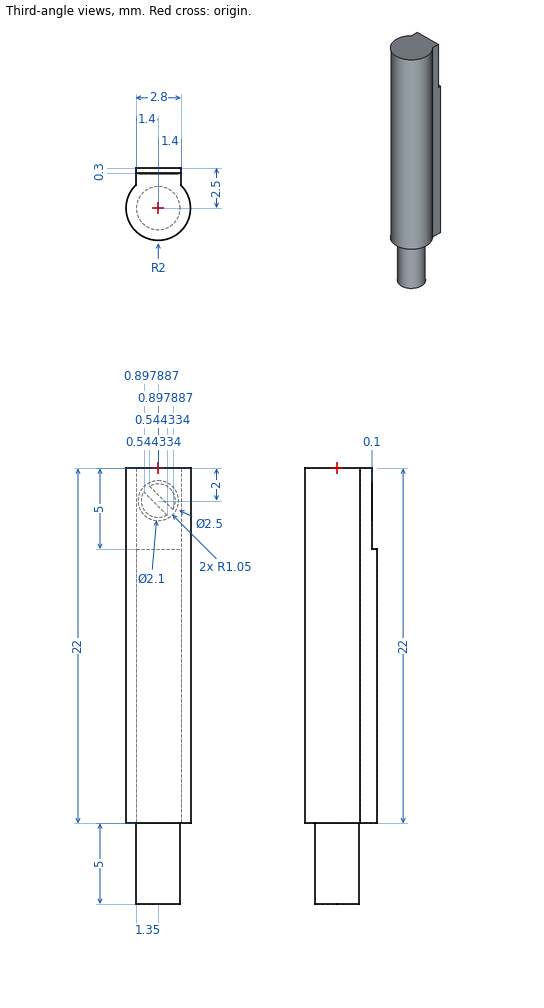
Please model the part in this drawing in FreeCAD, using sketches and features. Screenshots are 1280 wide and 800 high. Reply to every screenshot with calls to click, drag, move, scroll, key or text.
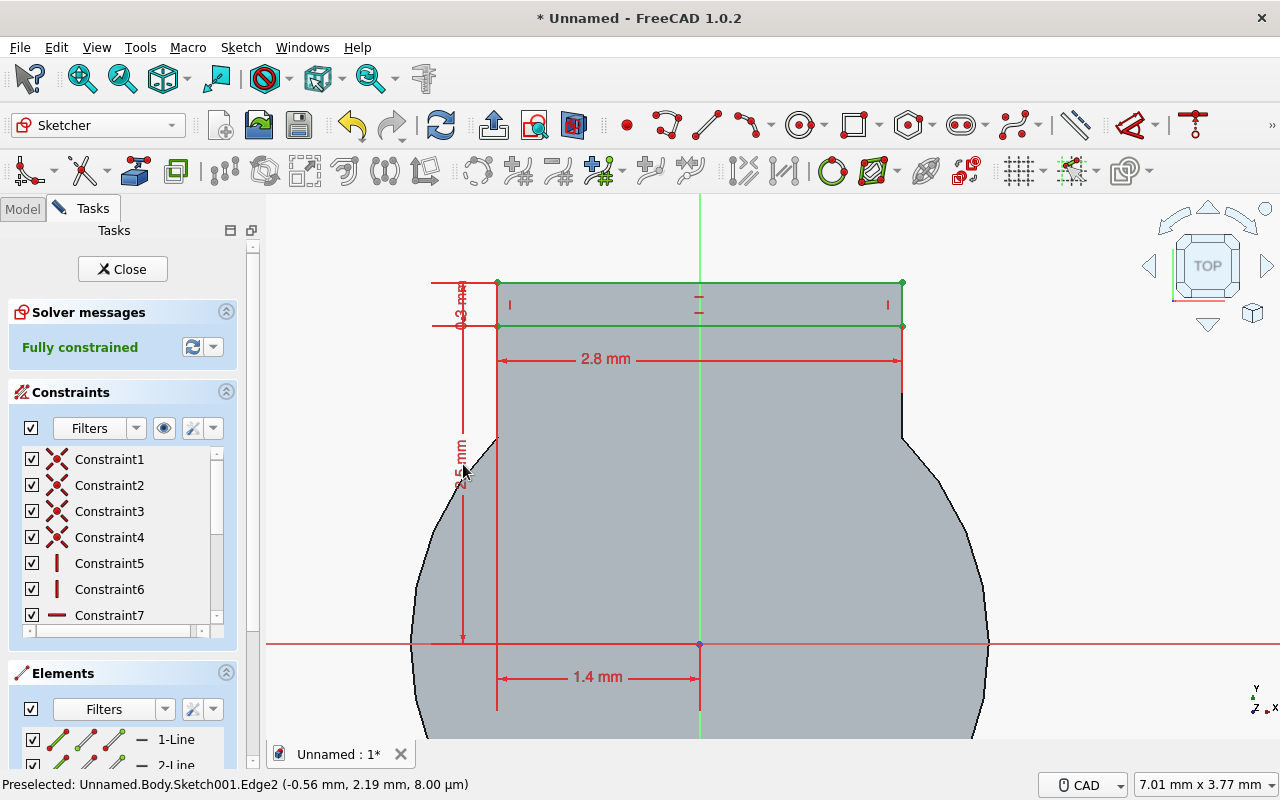
click(123, 269)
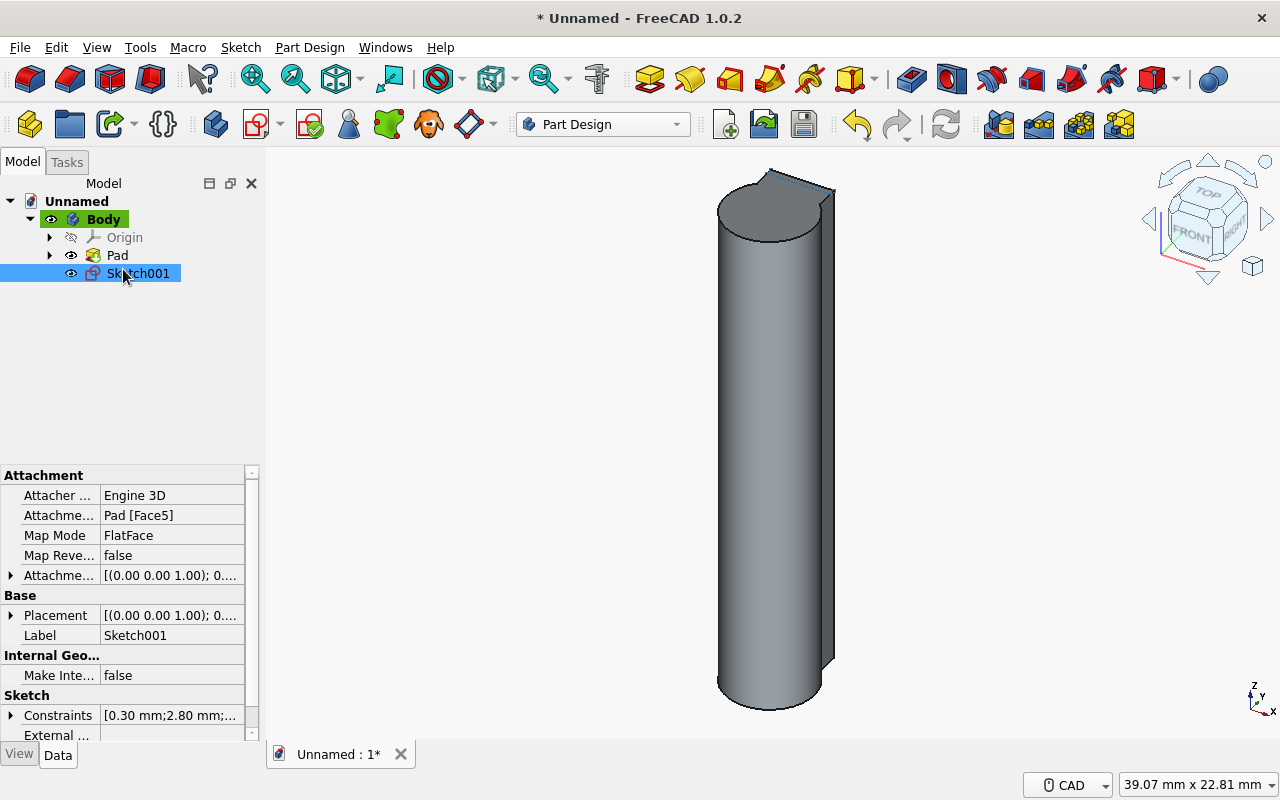
click(912, 80)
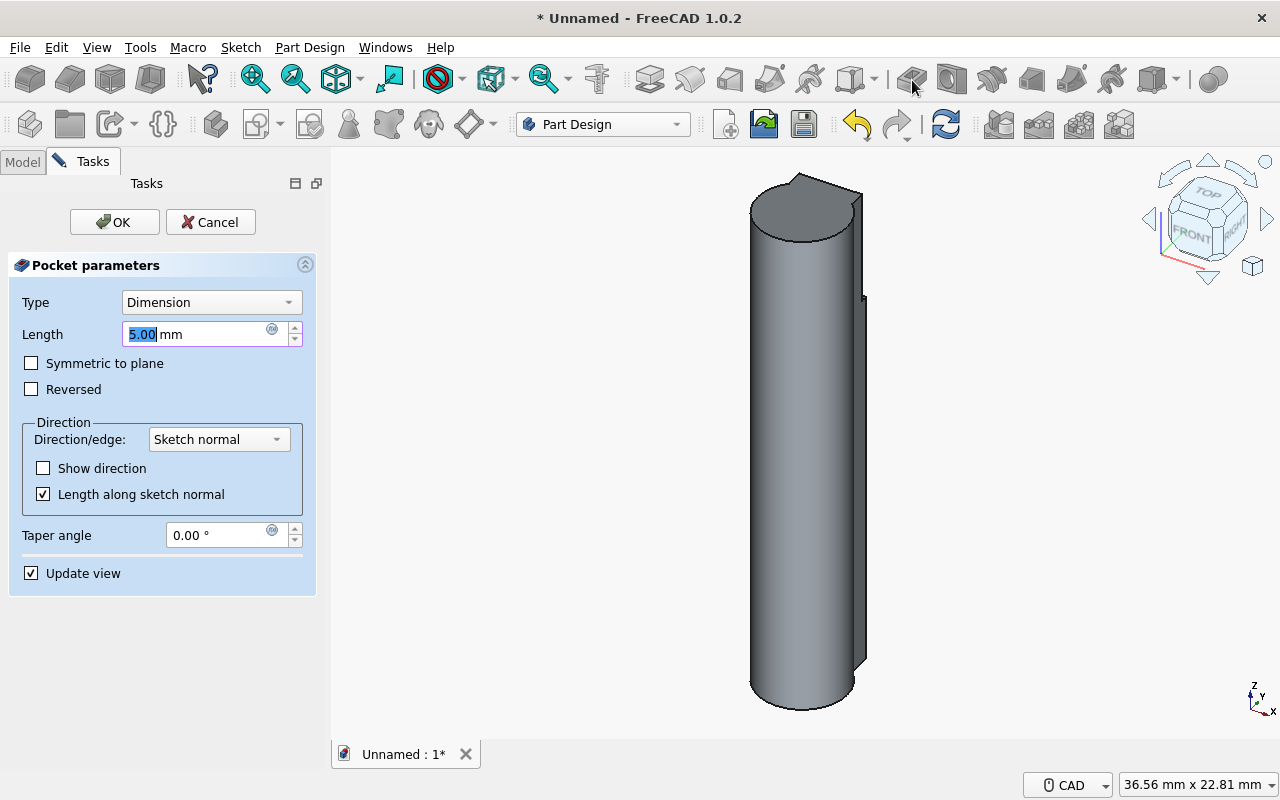
text(5)
key(Tab)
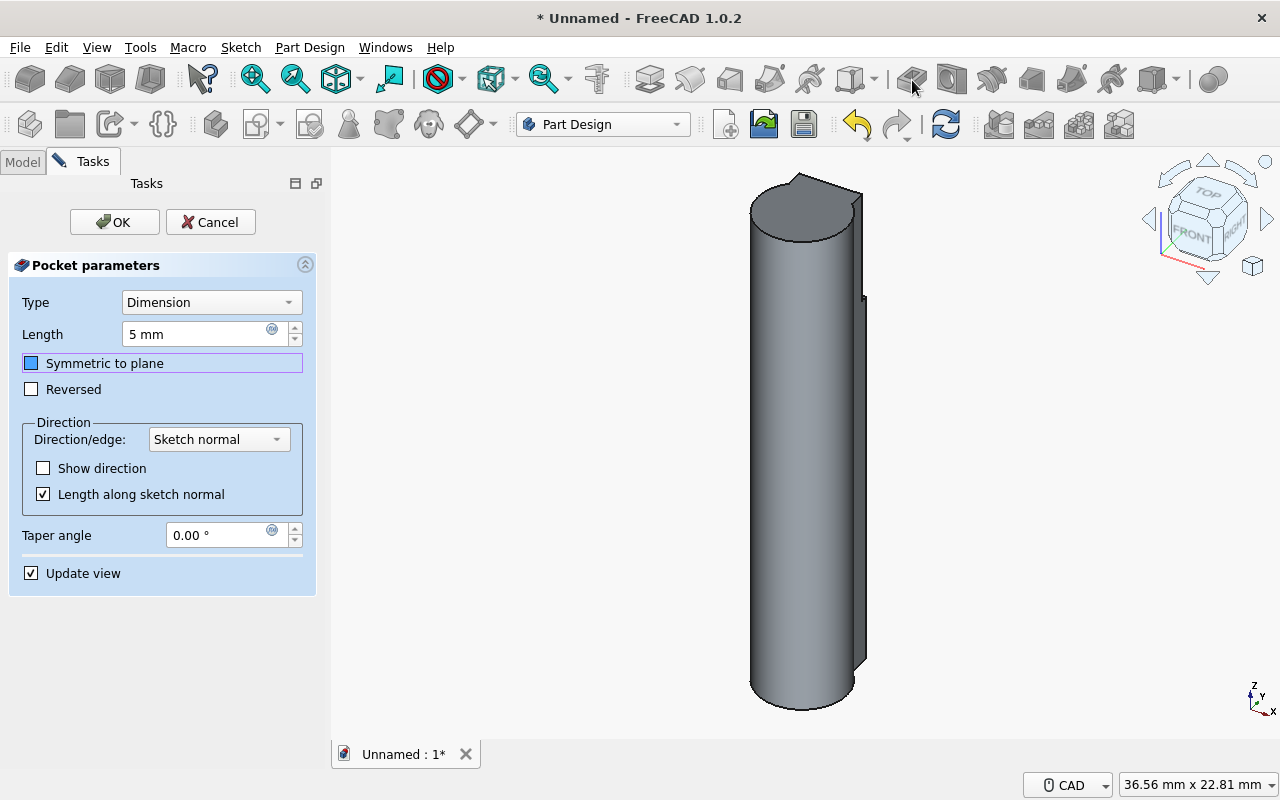
click(115, 222)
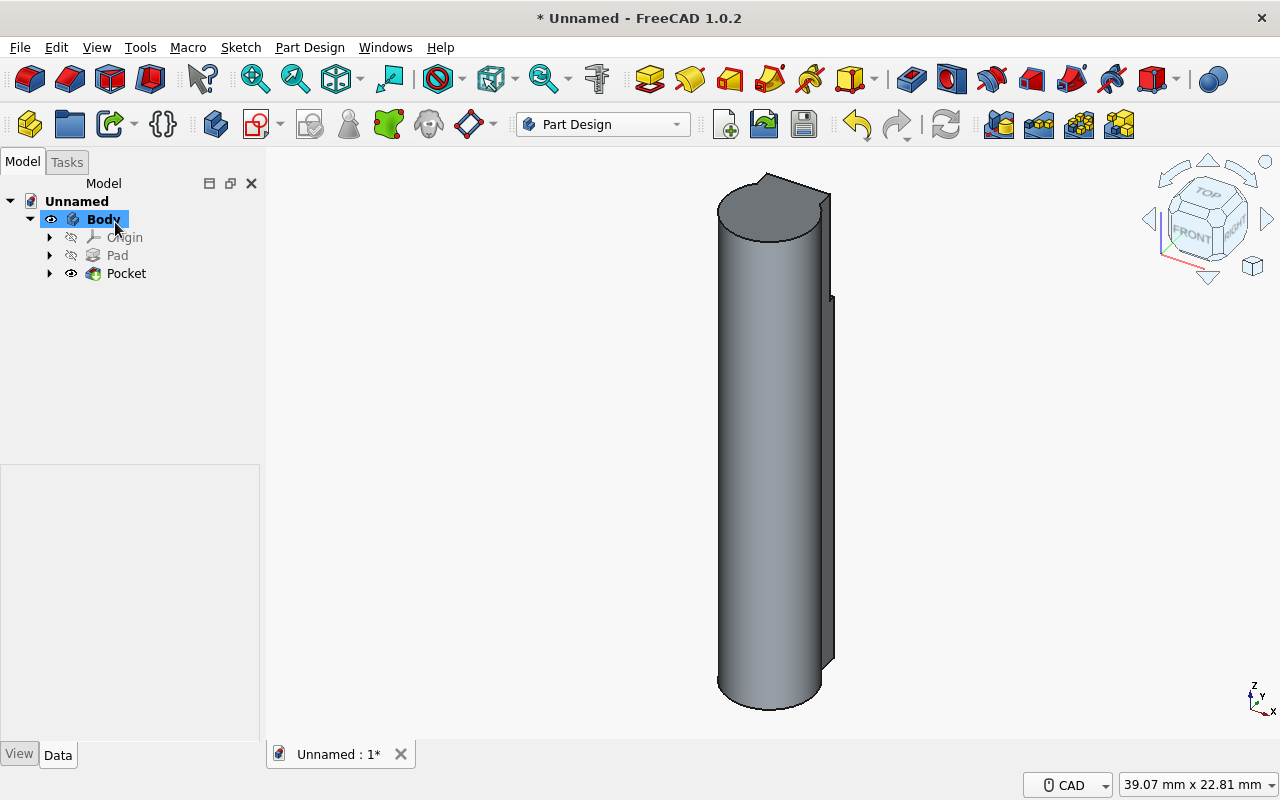
key(4)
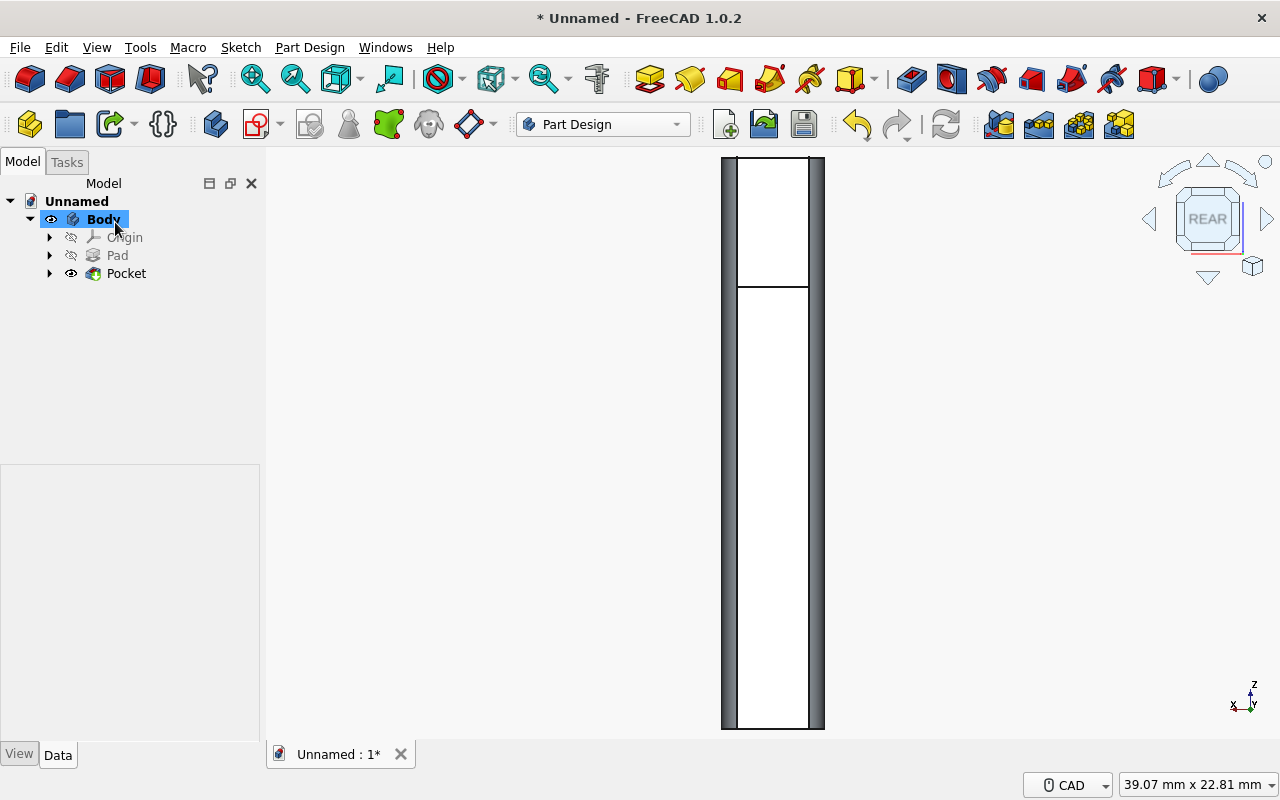
click(773, 203)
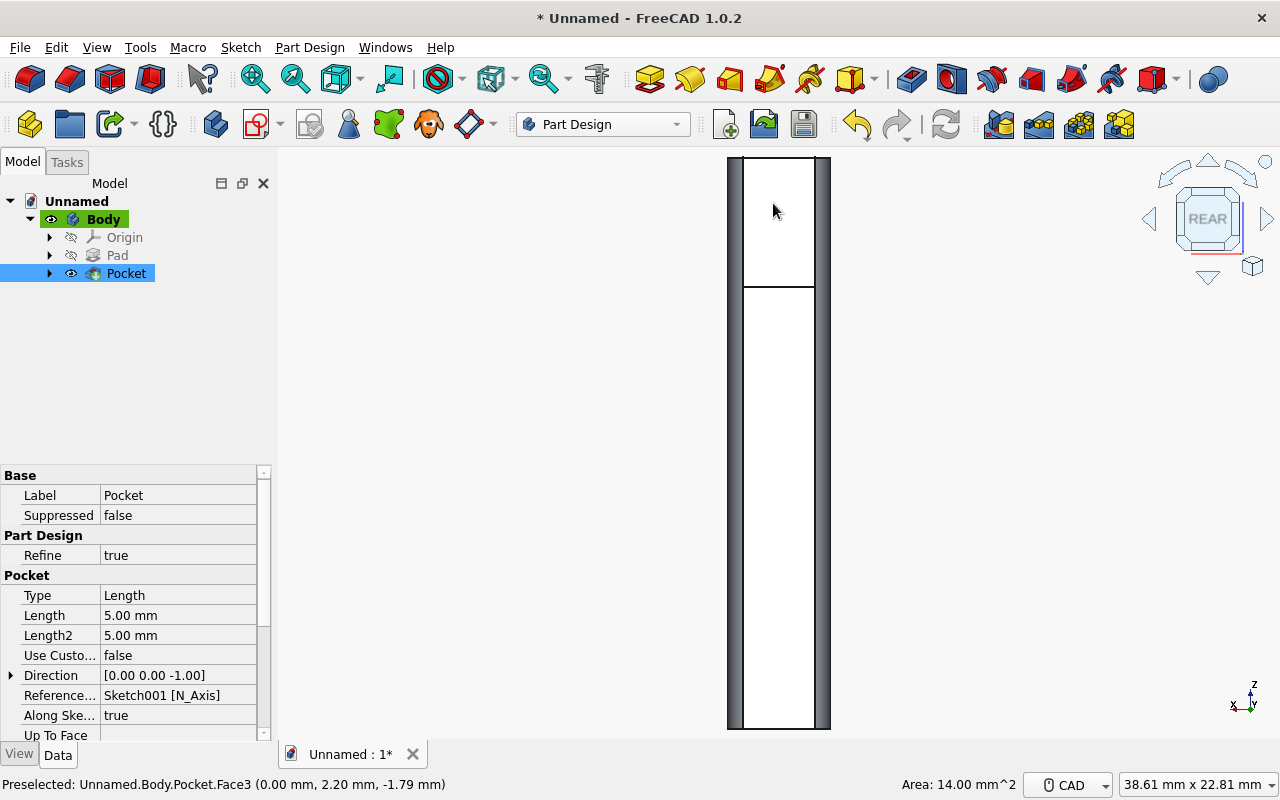
click(256, 124)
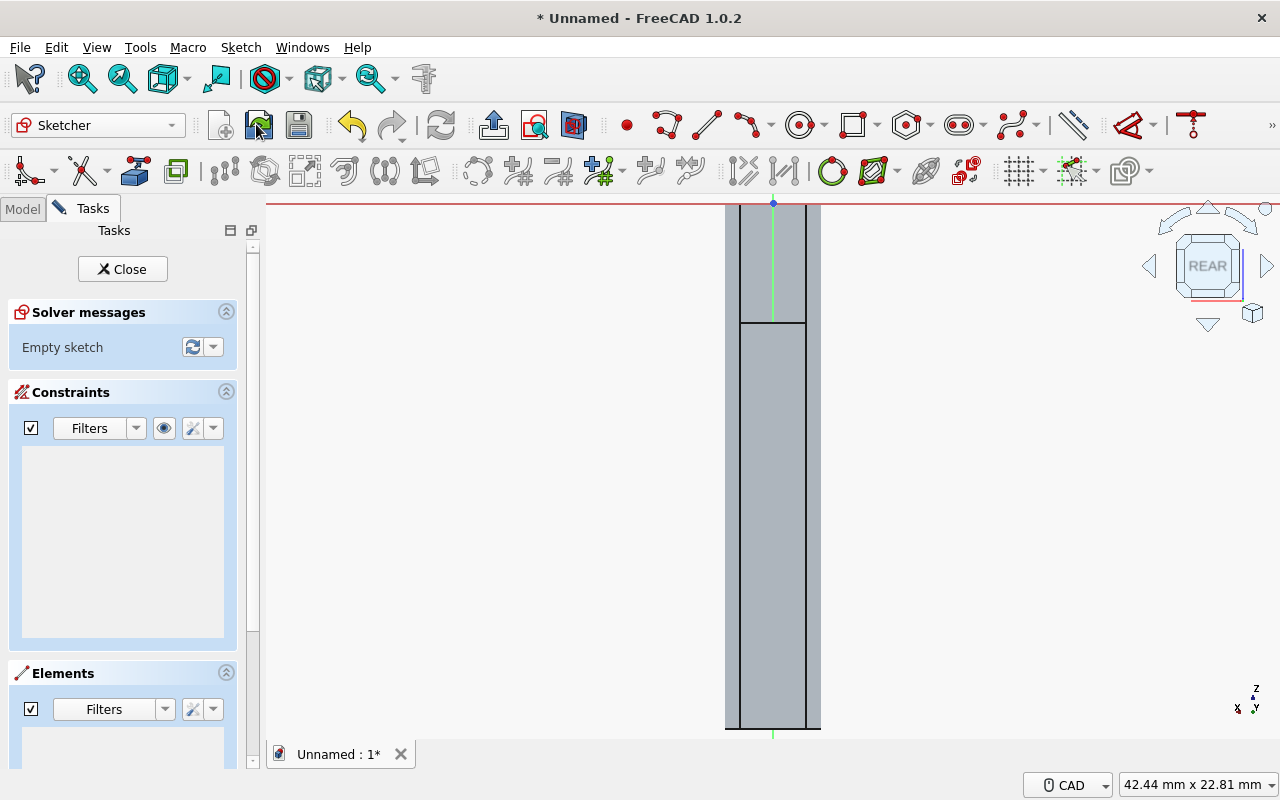
click(574, 126)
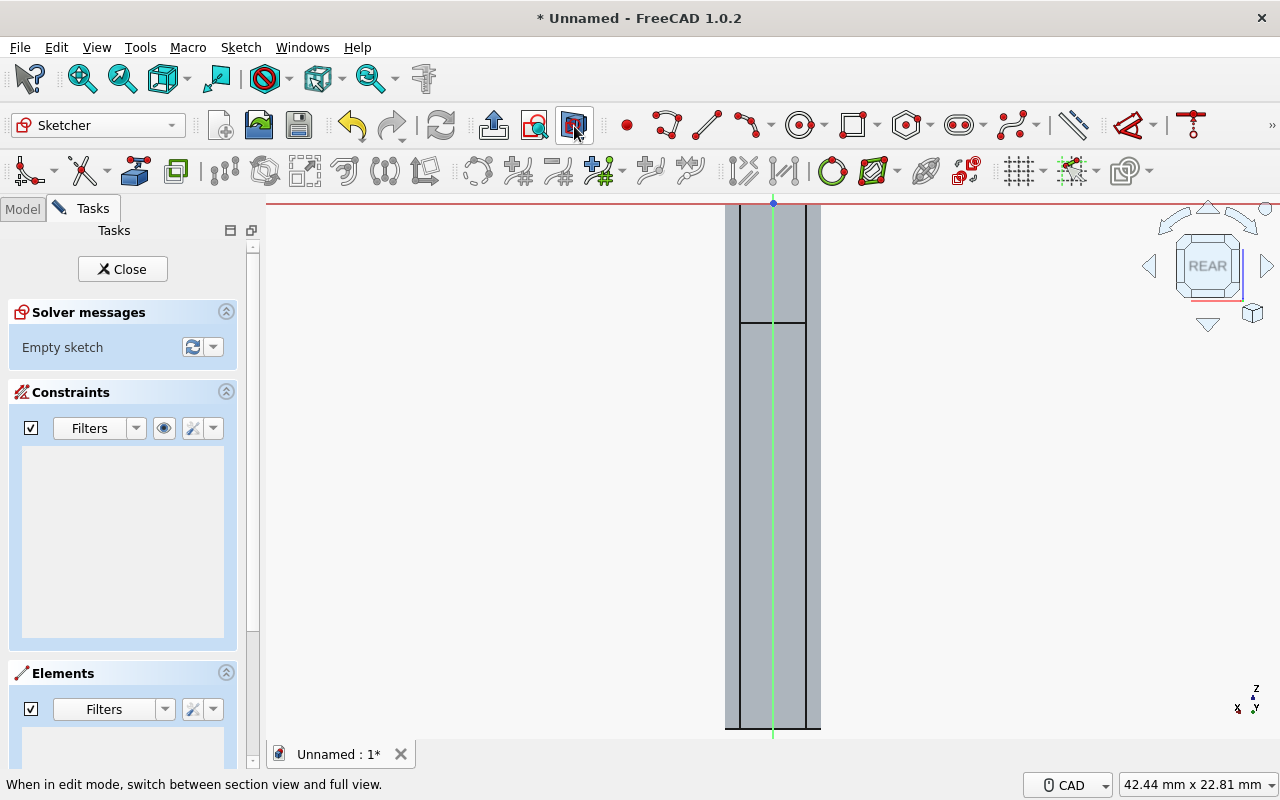
scroll(704, 466, down, 5)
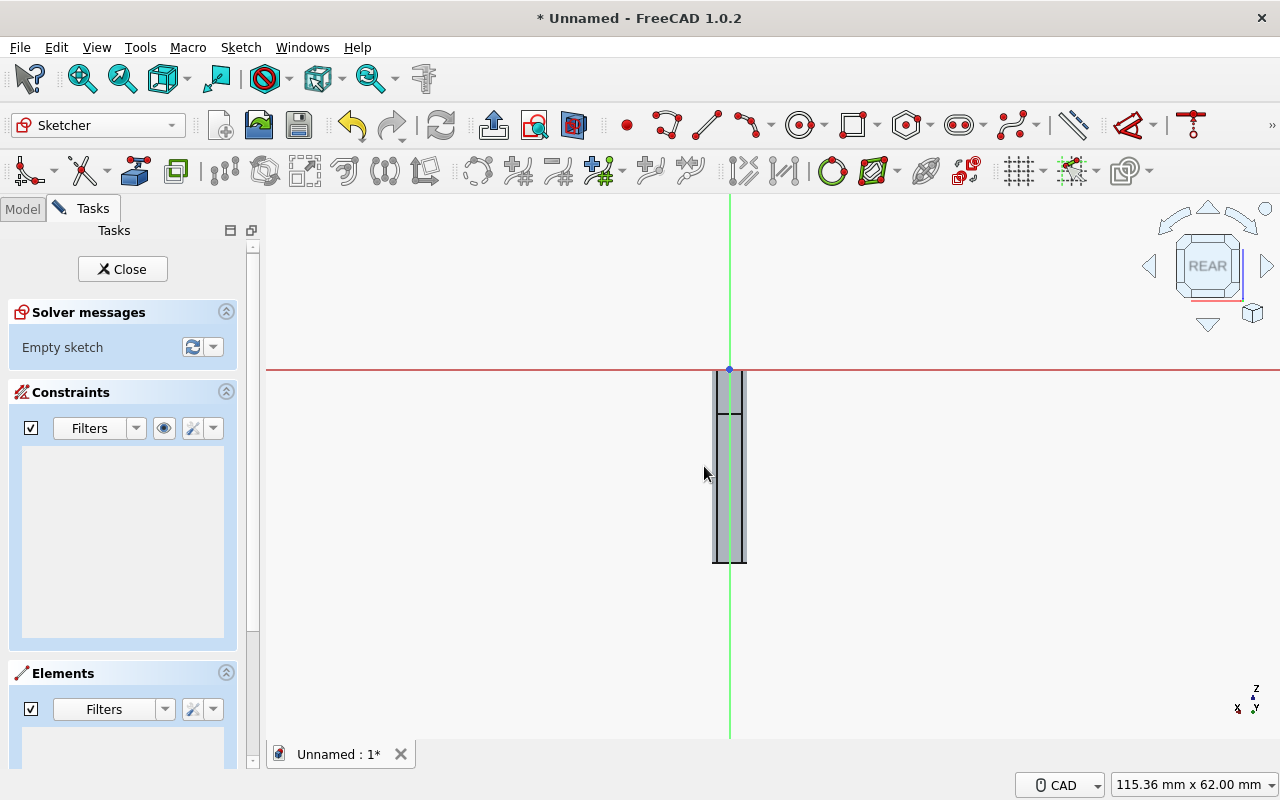
scroll(732, 376, up, 12)